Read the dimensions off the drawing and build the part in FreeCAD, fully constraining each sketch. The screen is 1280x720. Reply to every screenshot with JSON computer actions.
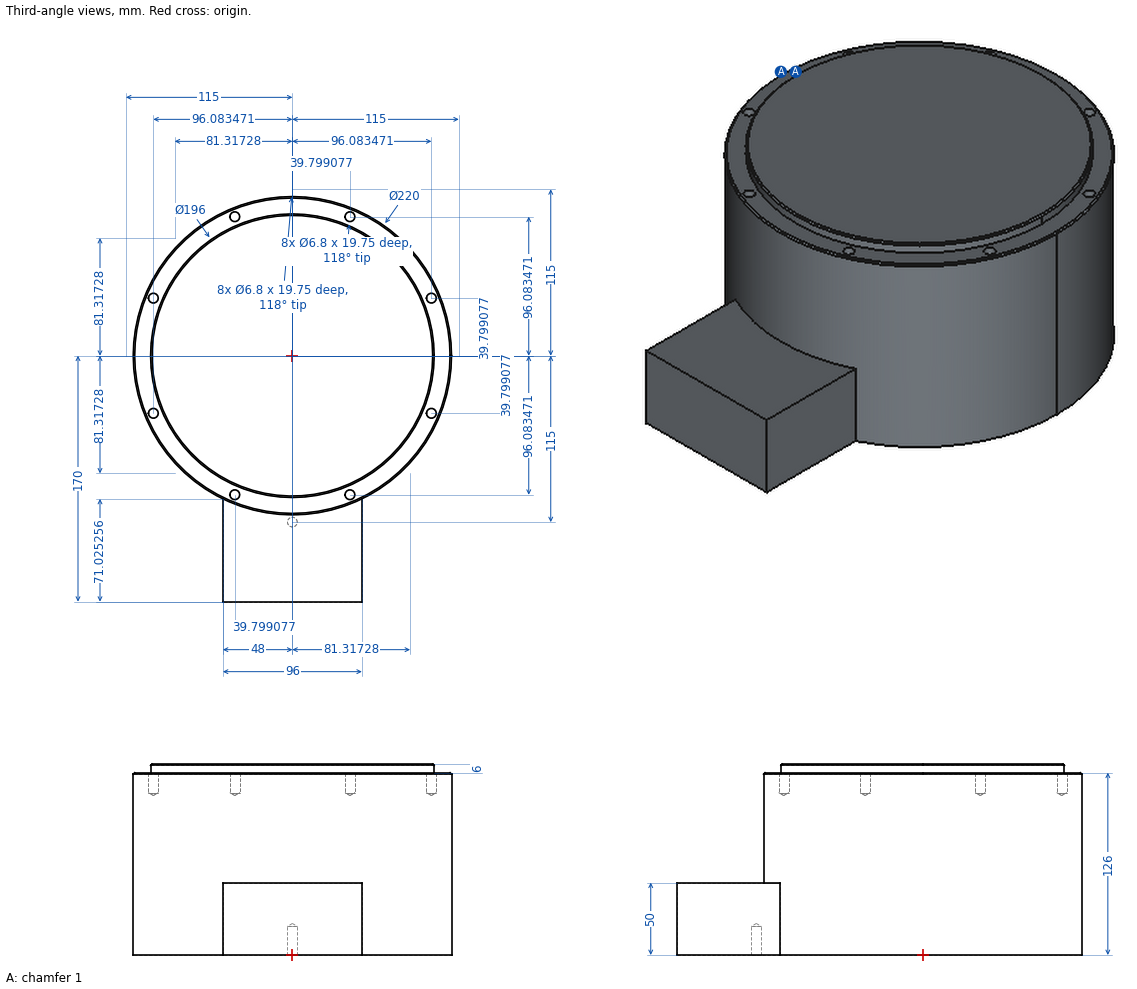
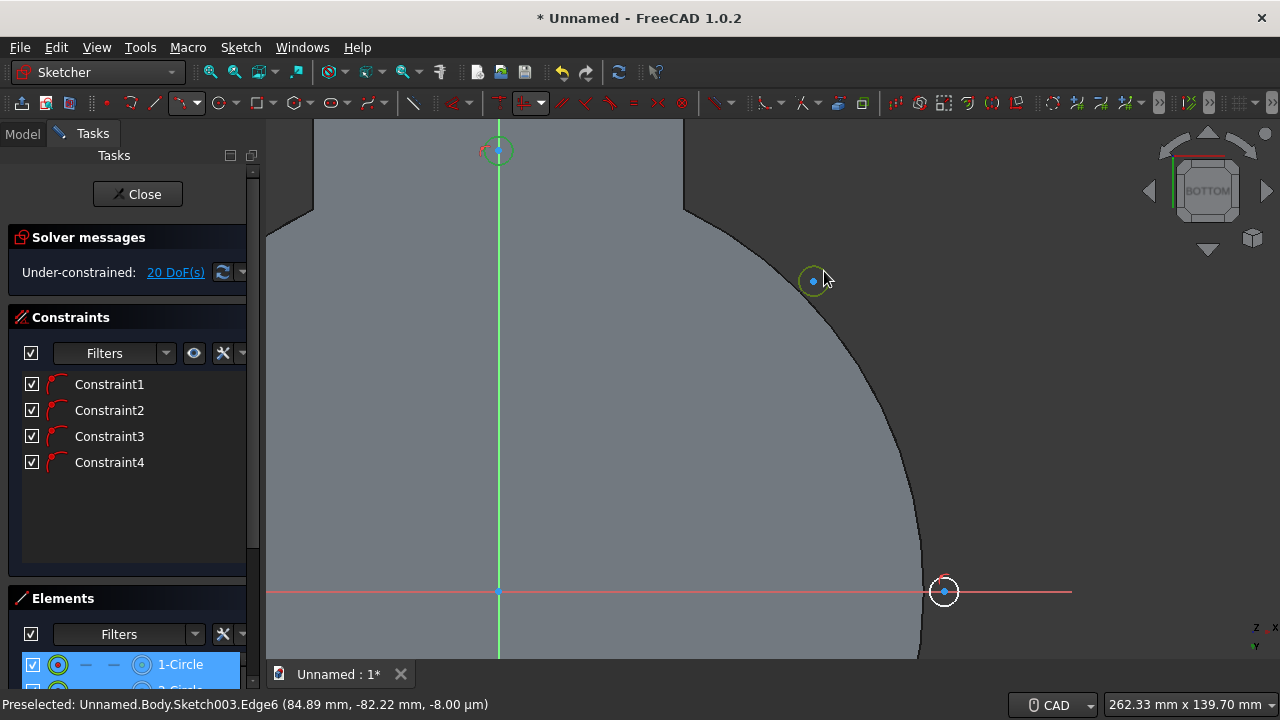
{"action": "scroll", "coordinate": [954, 582], "scroll_direction": "up", "scroll_amount": 2}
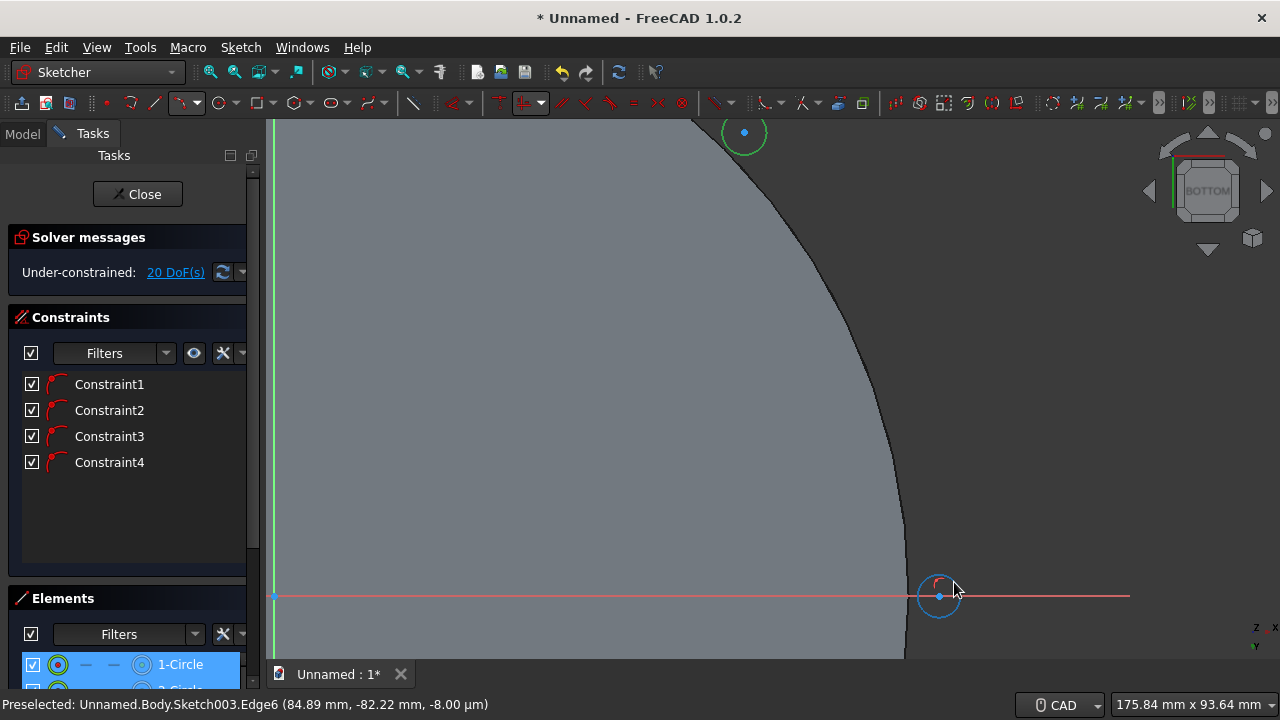
{"action": "left_click", "coordinate": [954, 581]}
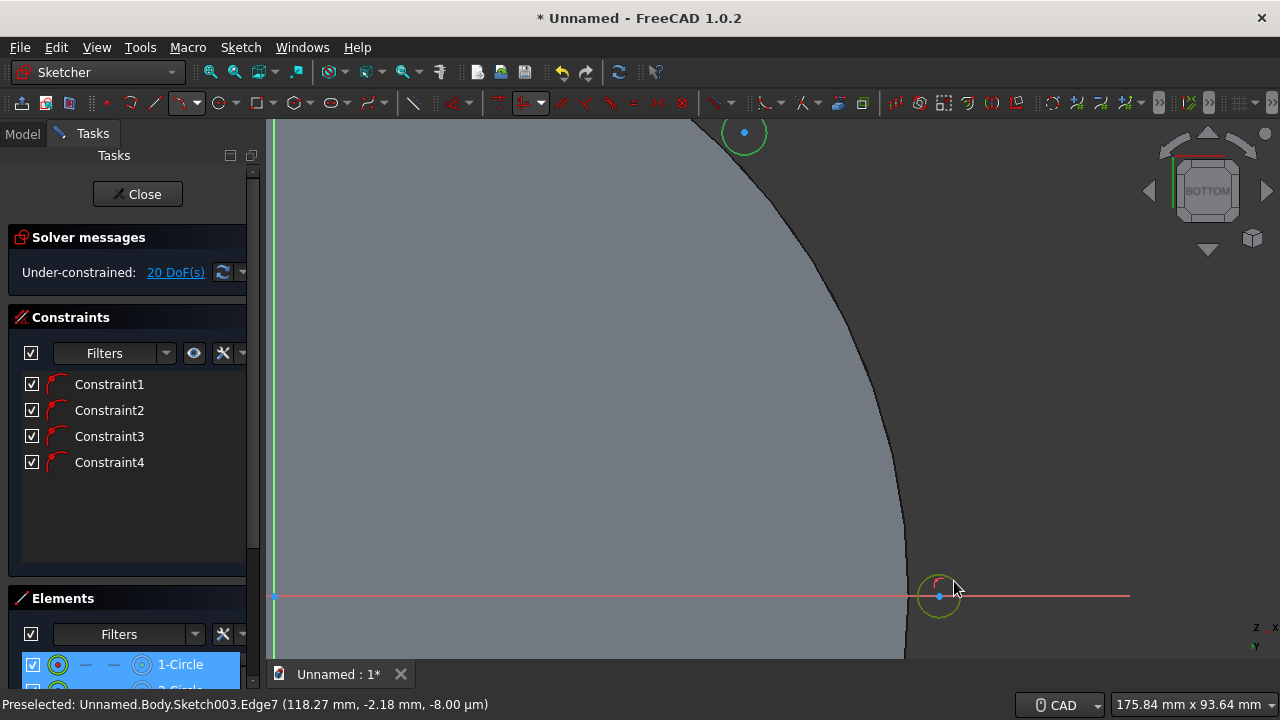
{"action": "scroll", "coordinate": [845, 321], "scroll_direction": "down", "scroll_amount": 7}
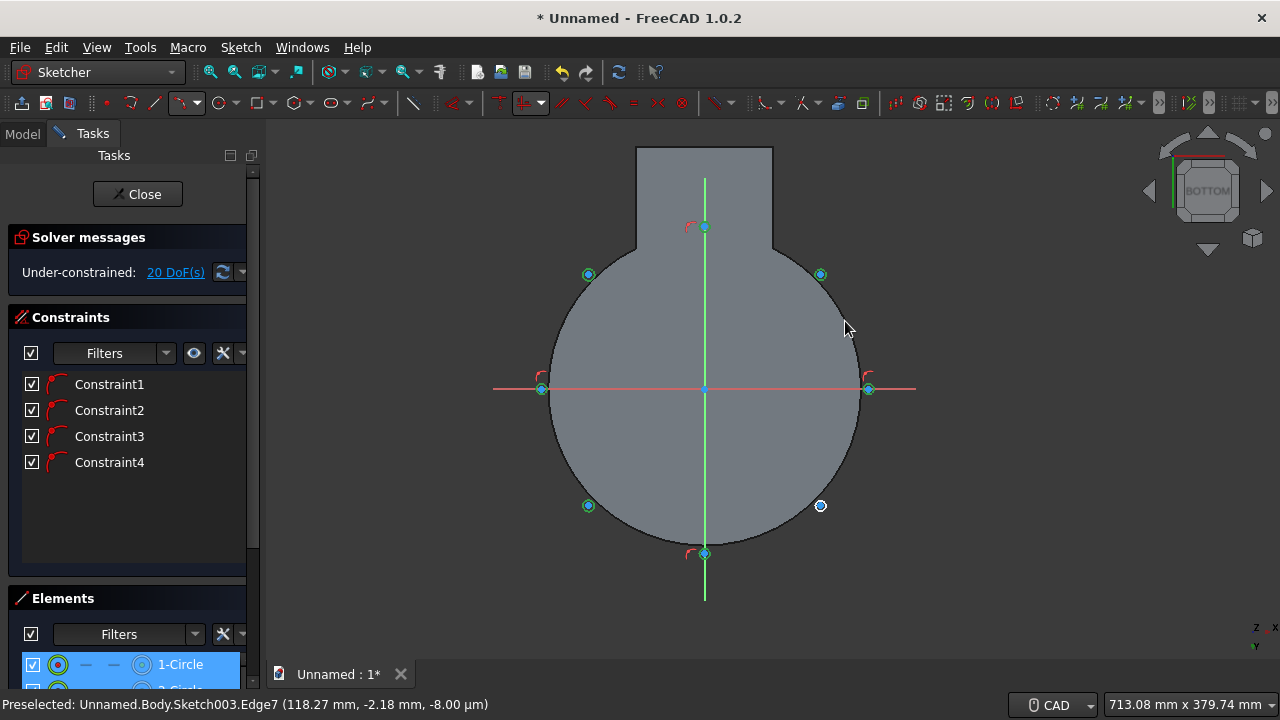
{"action": "scroll", "coordinate": [824, 502], "scroll_direction": "up", "scroll_amount": 5}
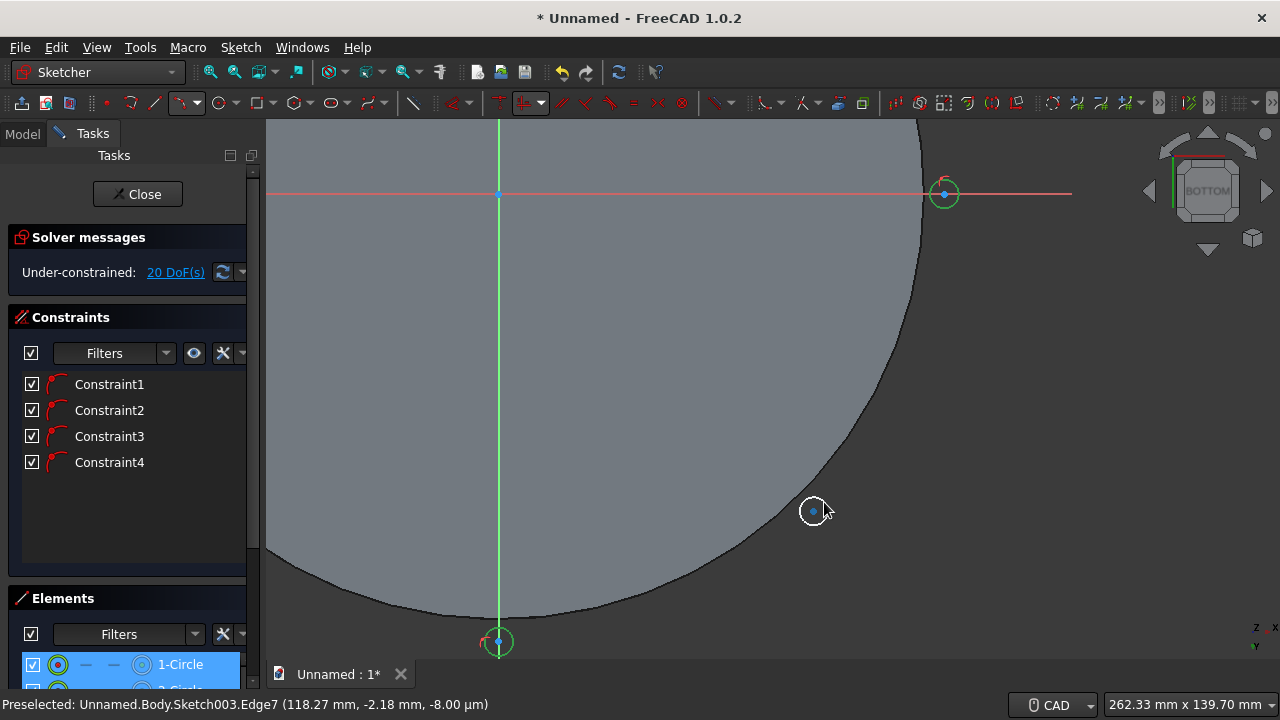
{"action": "left_click", "coordinate": [824, 501]}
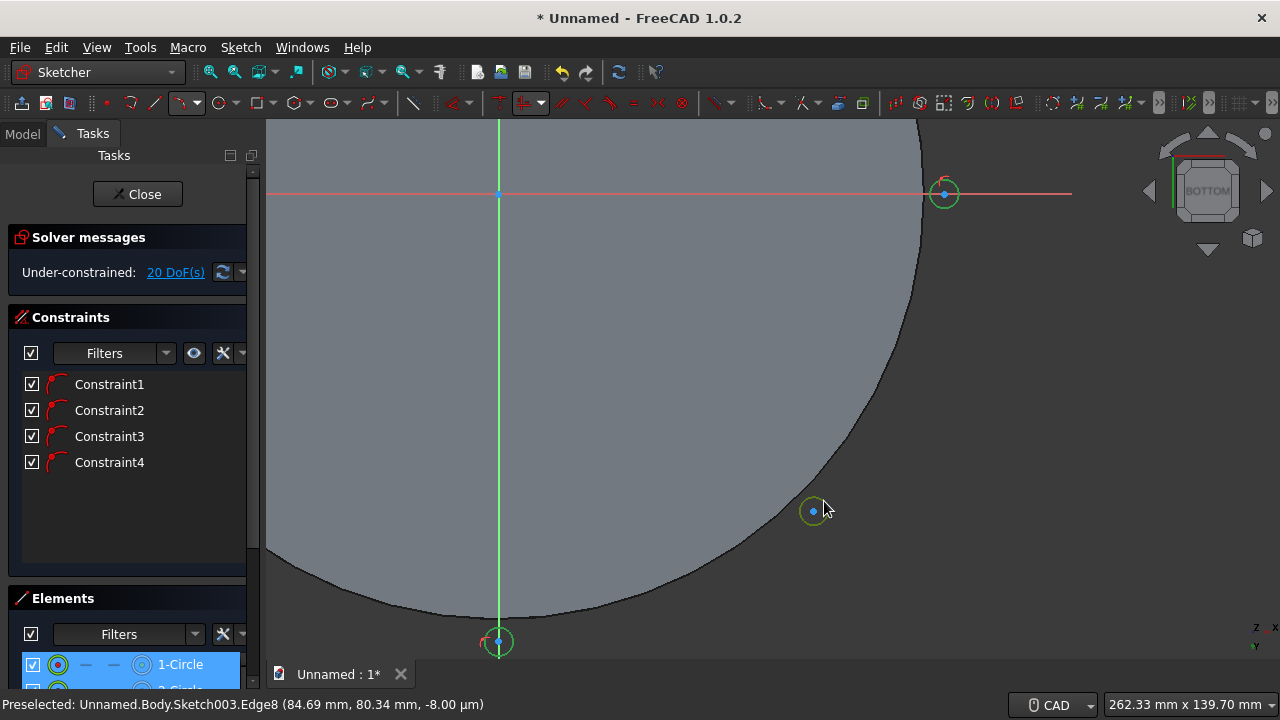
{"action": "left_click", "coordinate": [634, 104]}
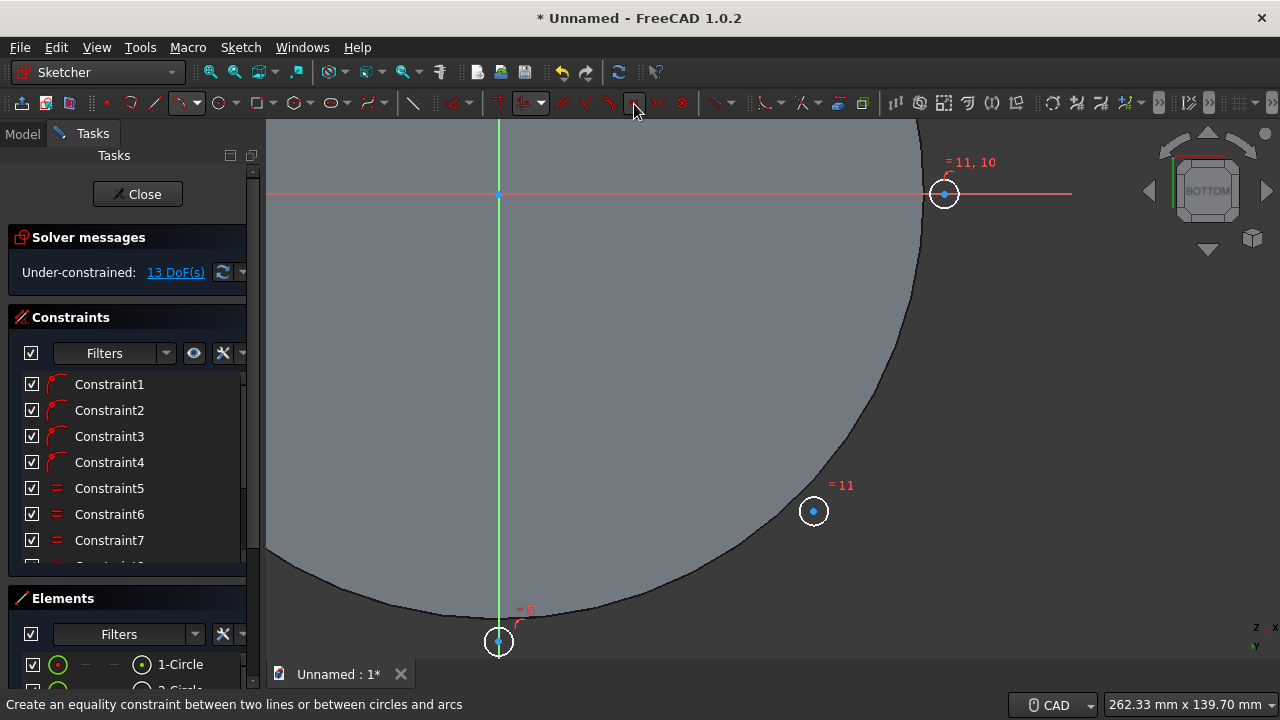
{"action": "scroll", "coordinate": [824, 502], "scroll_direction": "down", "scroll_amount": 5}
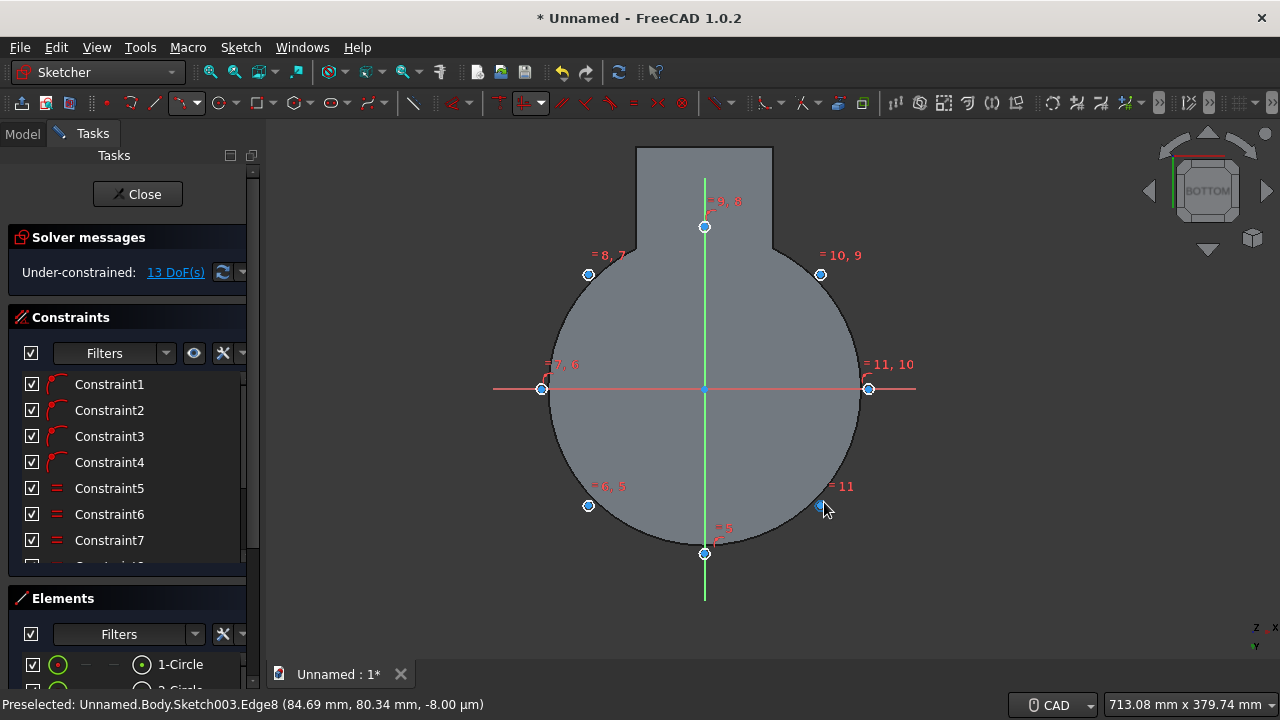
{"action": "left_click", "coordinate": [589, 506]}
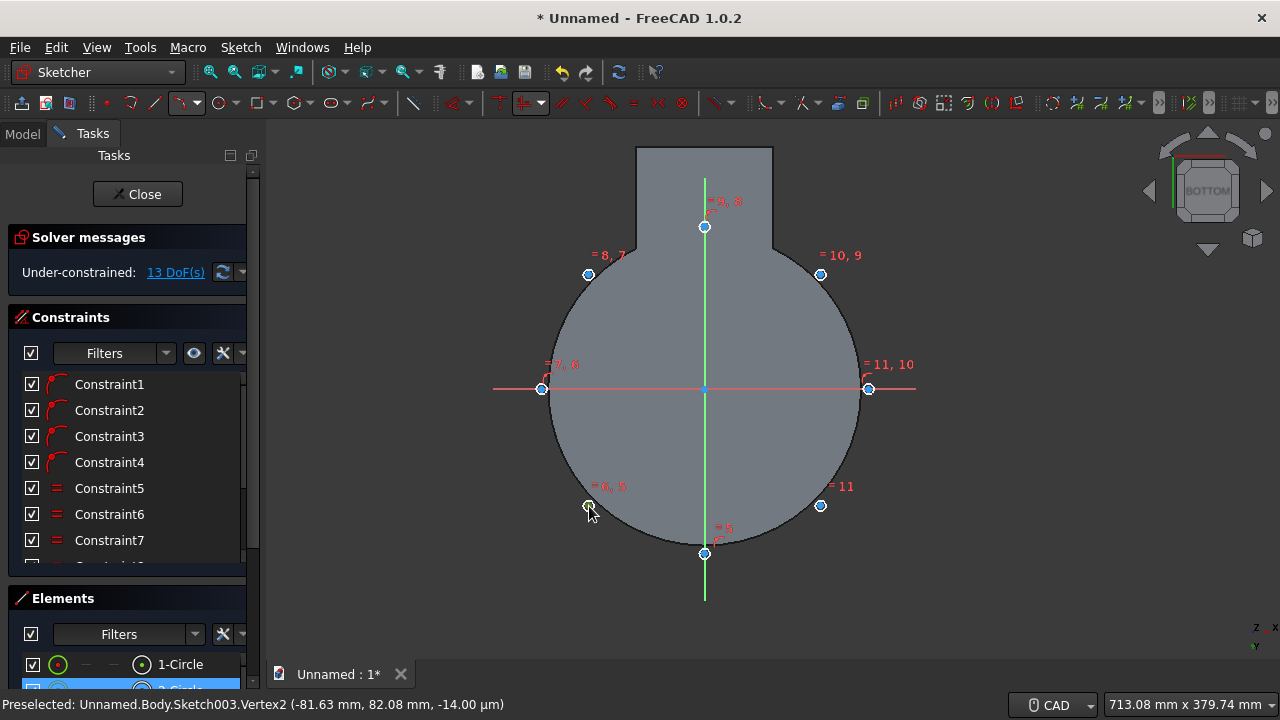
{"action": "left_click", "coordinate": [589, 275]}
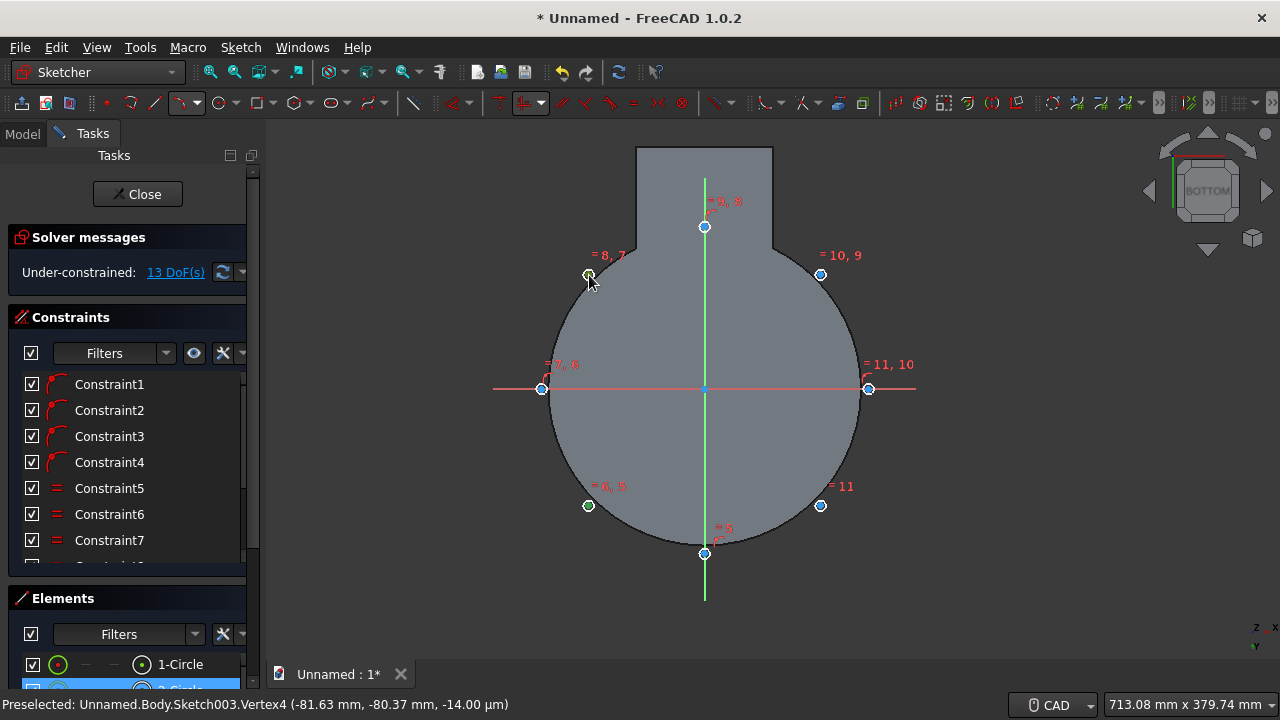
{"action": "left_click", "coordinate": [544, 104]}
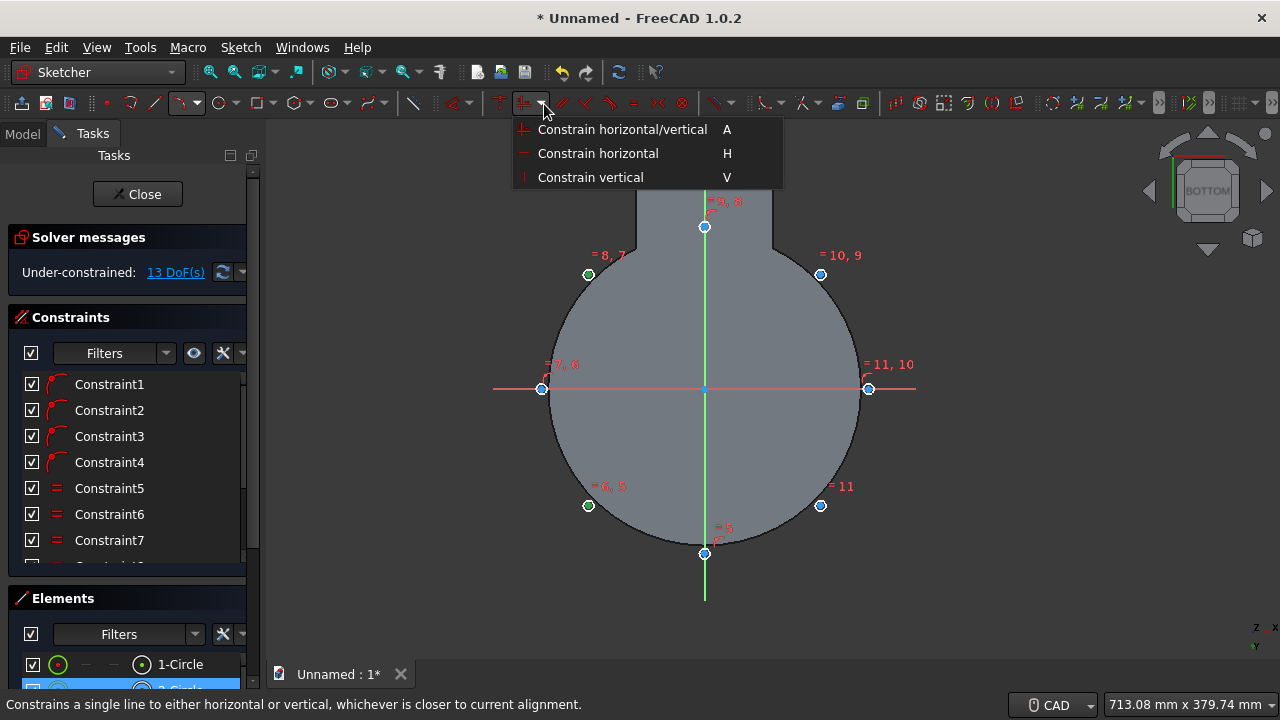
{"action": "left_click", "coordinate": [648, 177]}